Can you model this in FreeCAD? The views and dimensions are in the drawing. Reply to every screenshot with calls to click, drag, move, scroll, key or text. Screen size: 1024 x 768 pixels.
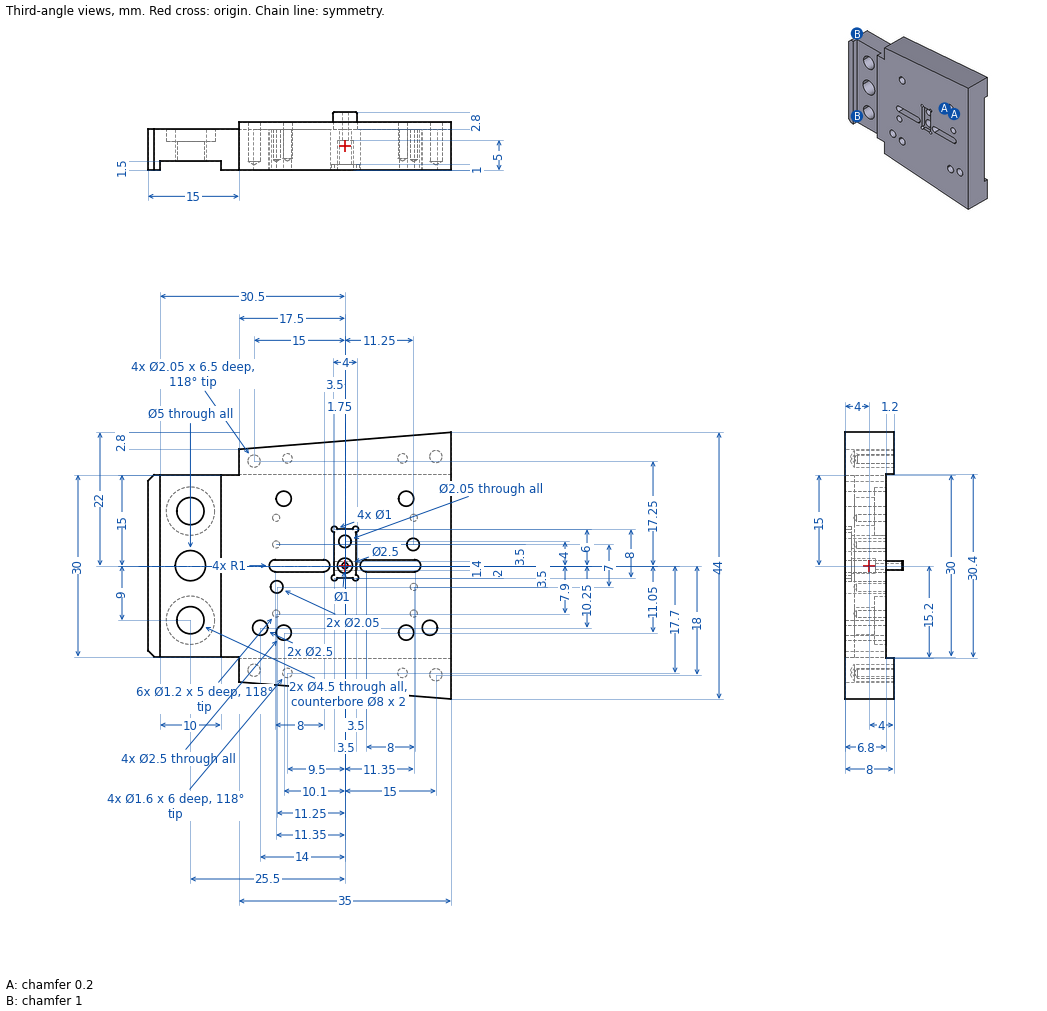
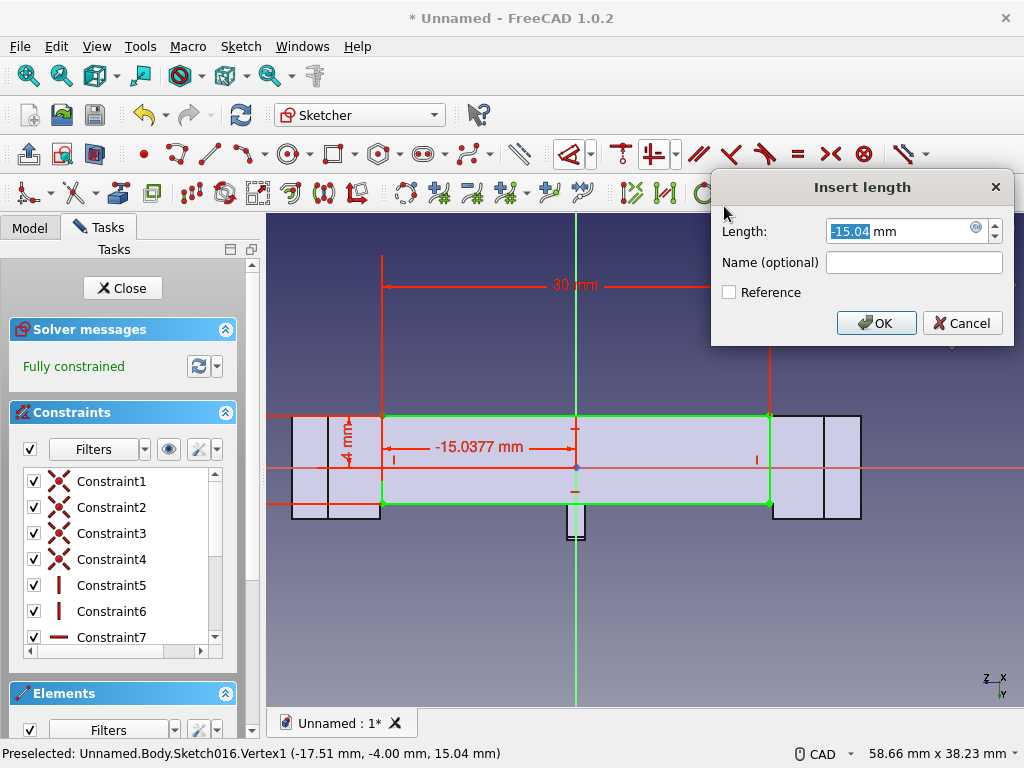
text(-15)
key(Return)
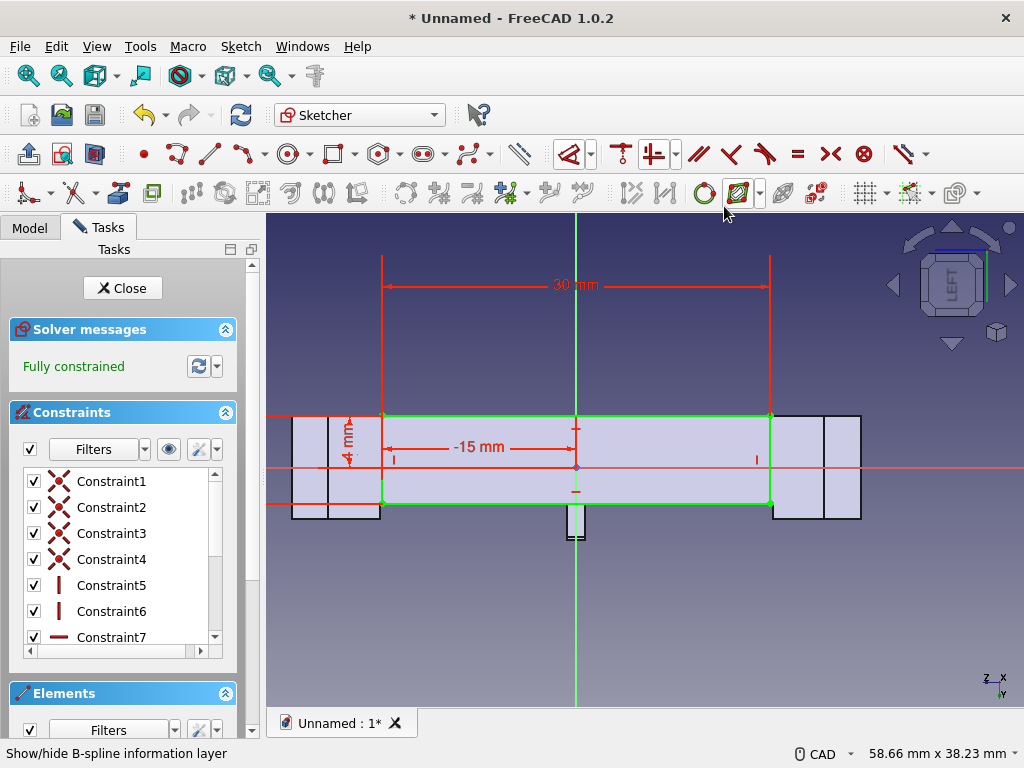
click(123, 288)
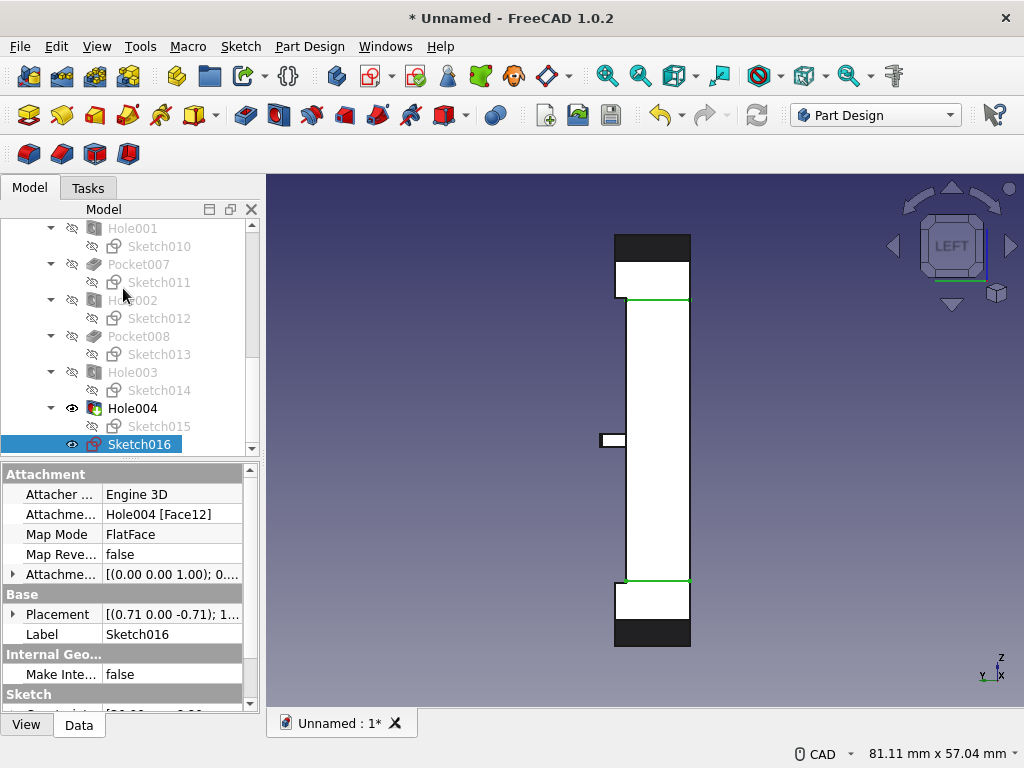
click(29, 116)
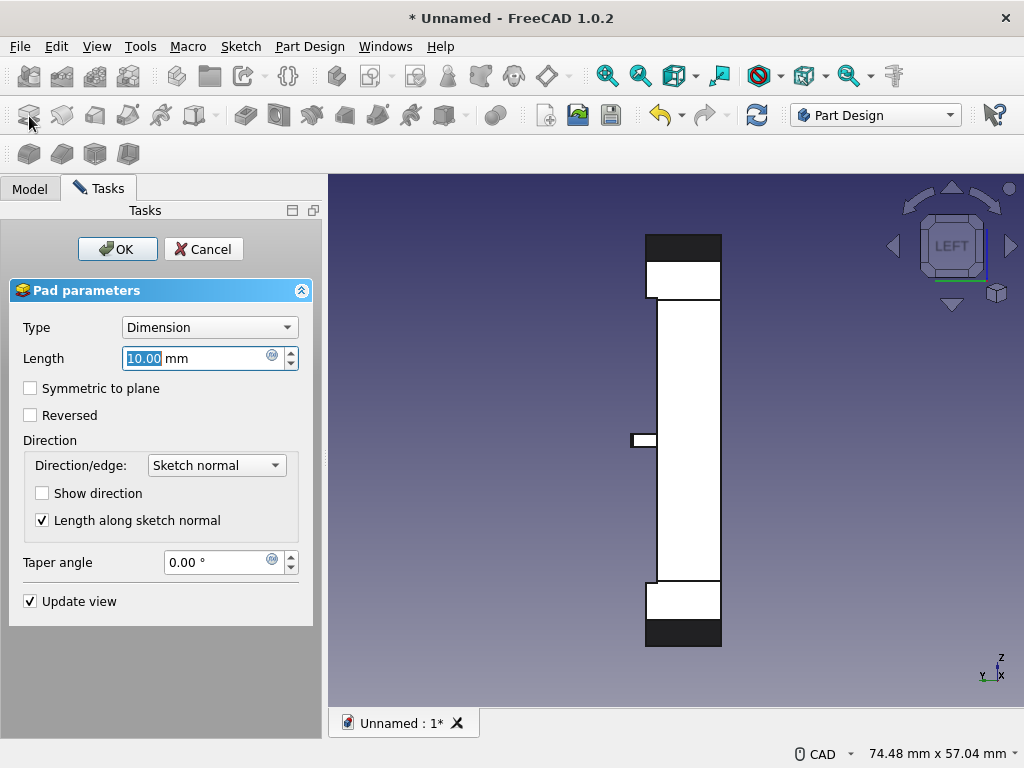
text(15)
key(Tab)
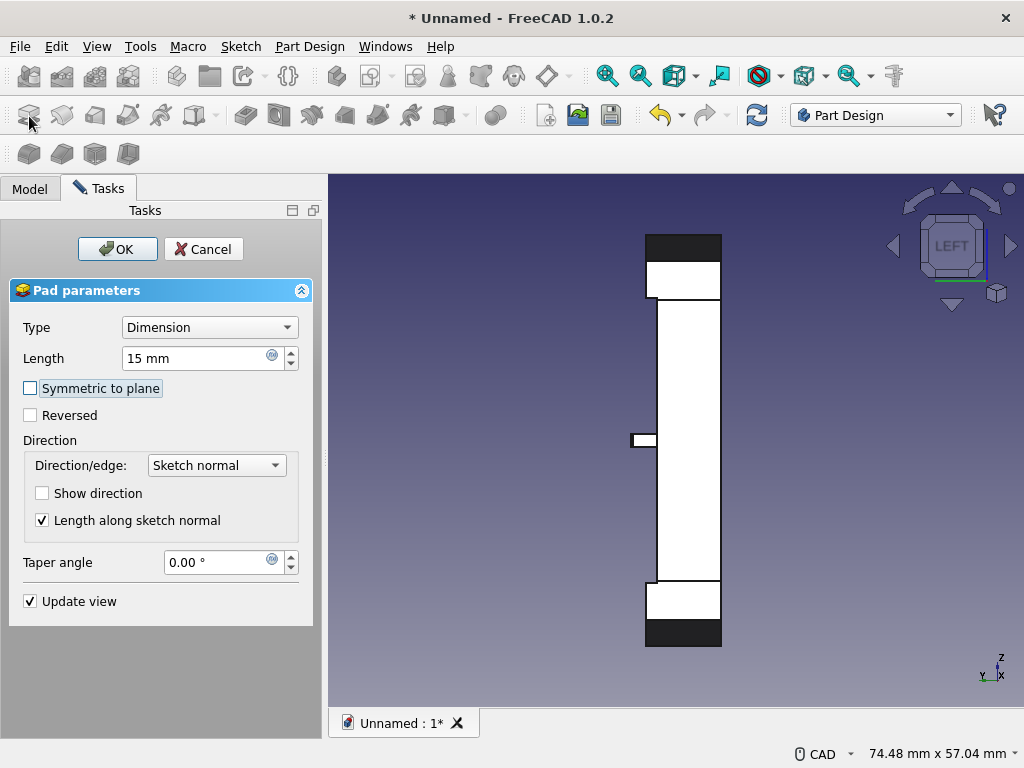
click(118, 249)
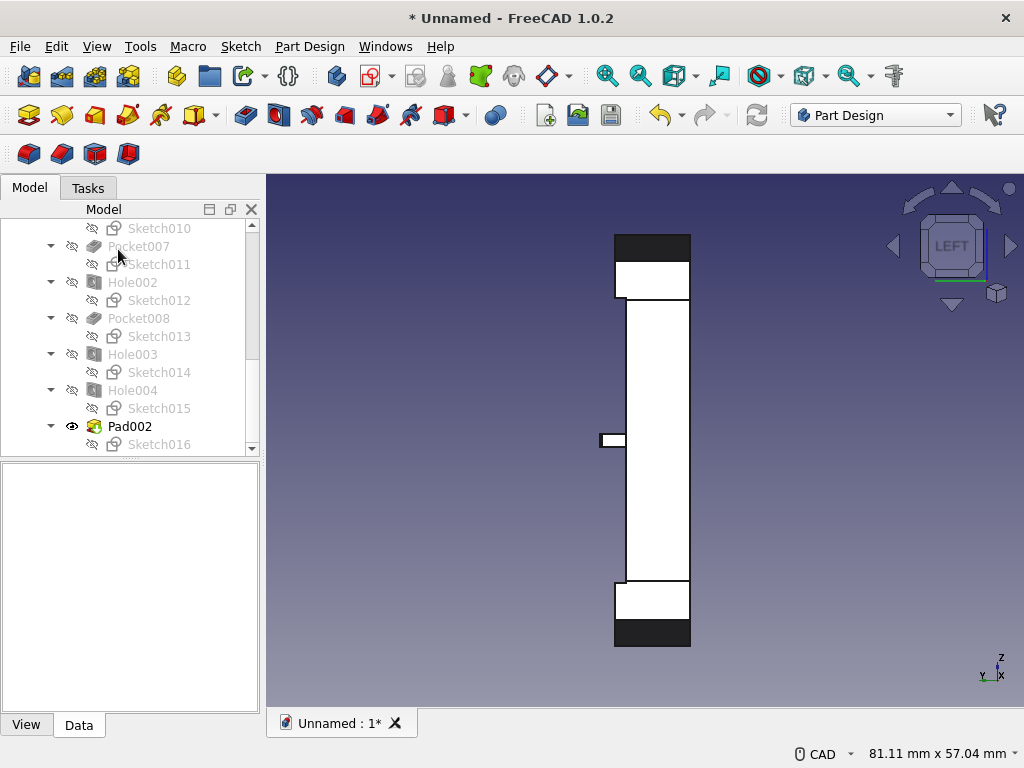
key(0)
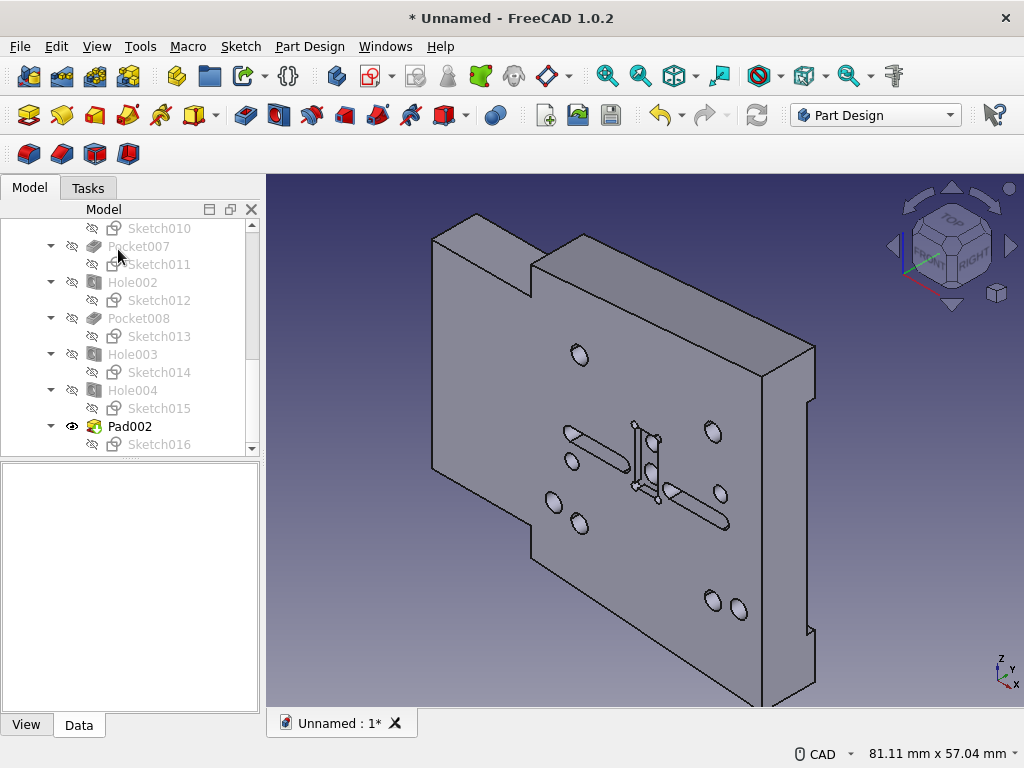
click(608, 76)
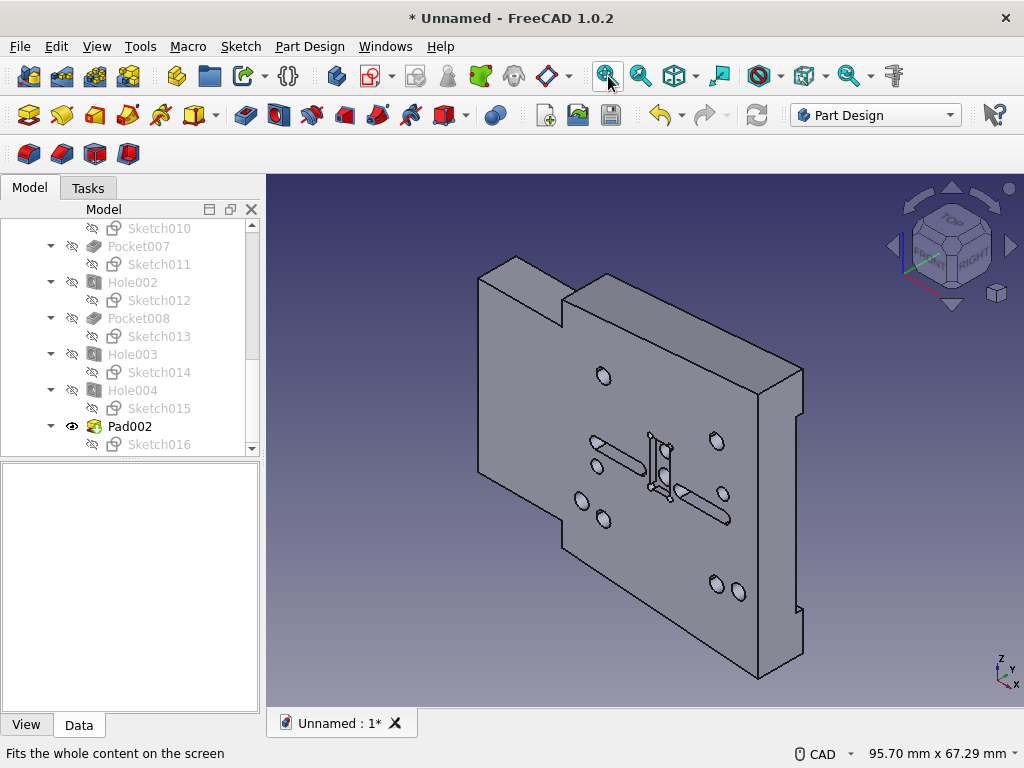
click(538, 409)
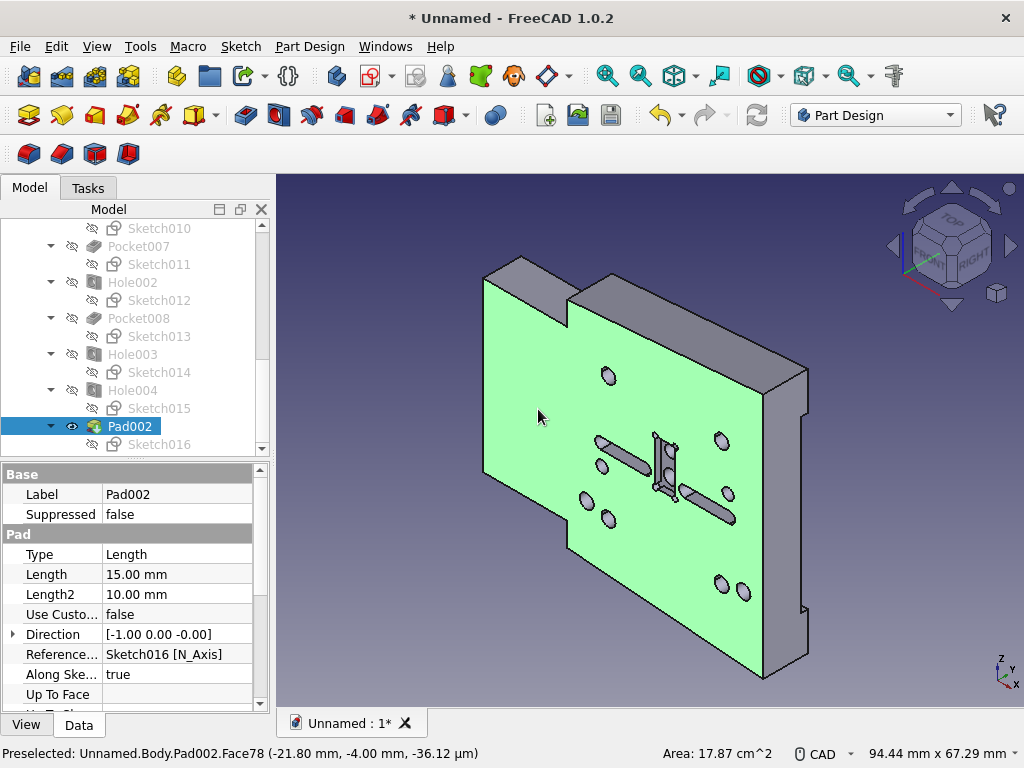
click(370, 76)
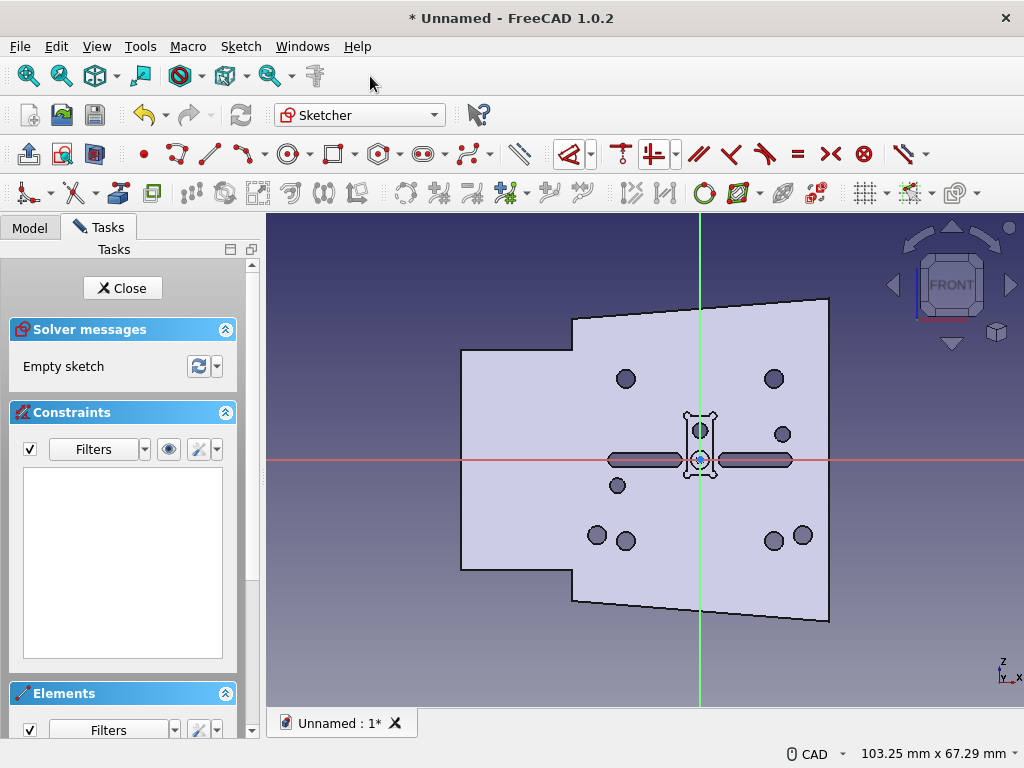
scroll(612, 460, up, 2)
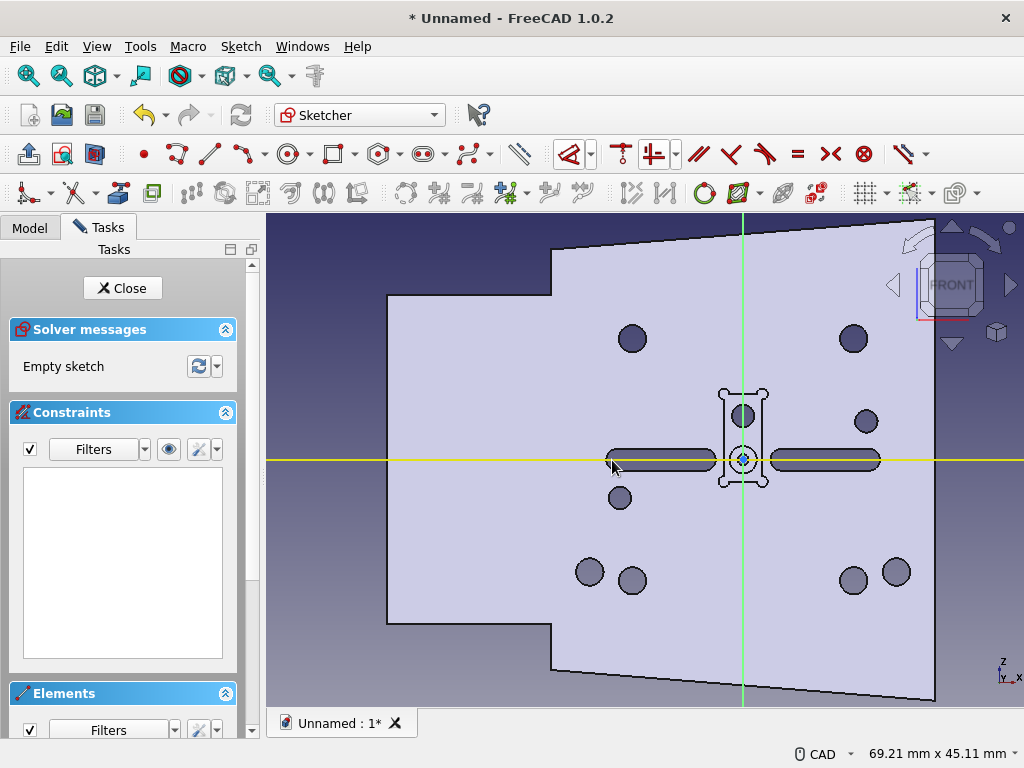
click(332, 154)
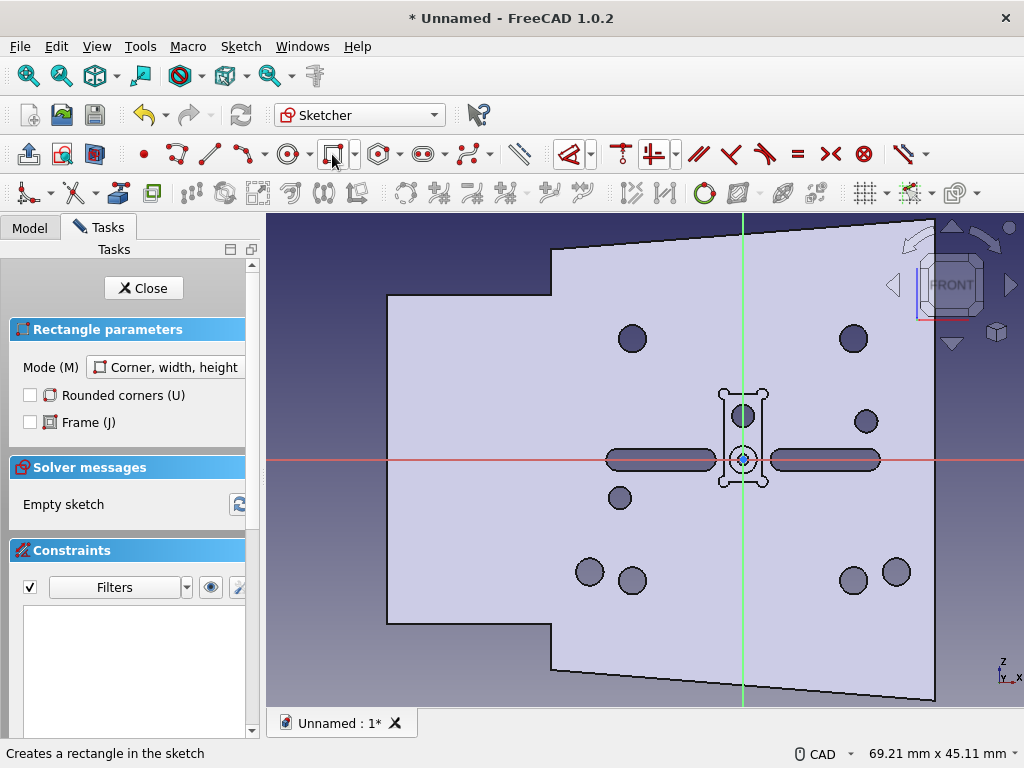
click(409, 295)
move(519, 624)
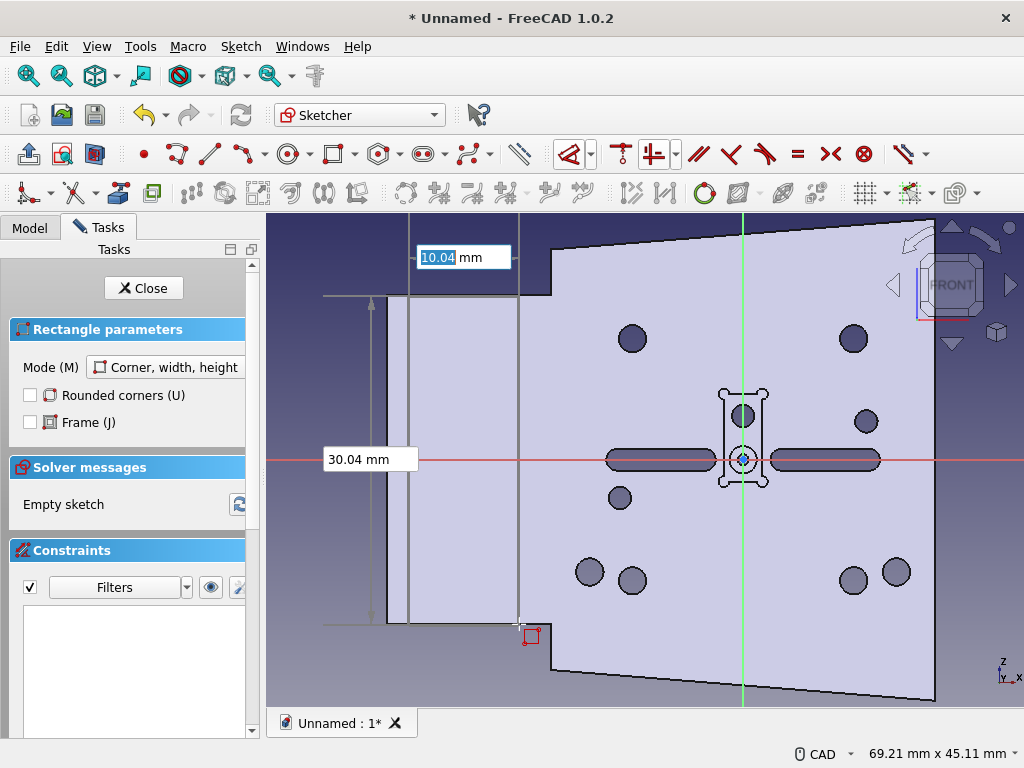
text(10)
key(Tab)
text(30)
key(Return)
key(Escape)